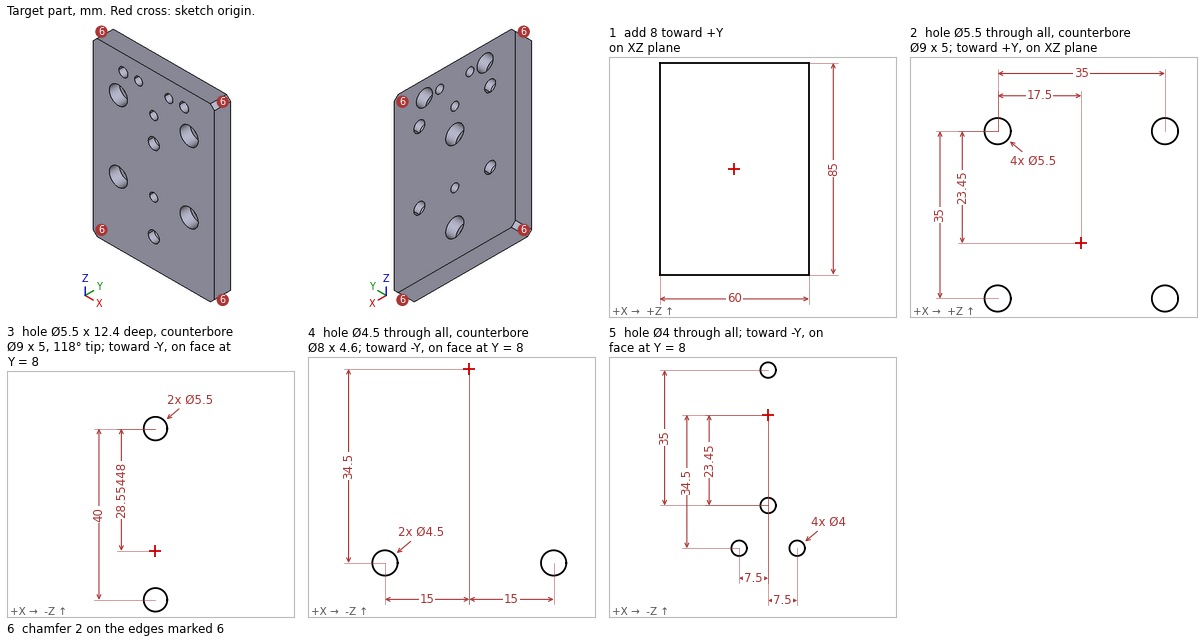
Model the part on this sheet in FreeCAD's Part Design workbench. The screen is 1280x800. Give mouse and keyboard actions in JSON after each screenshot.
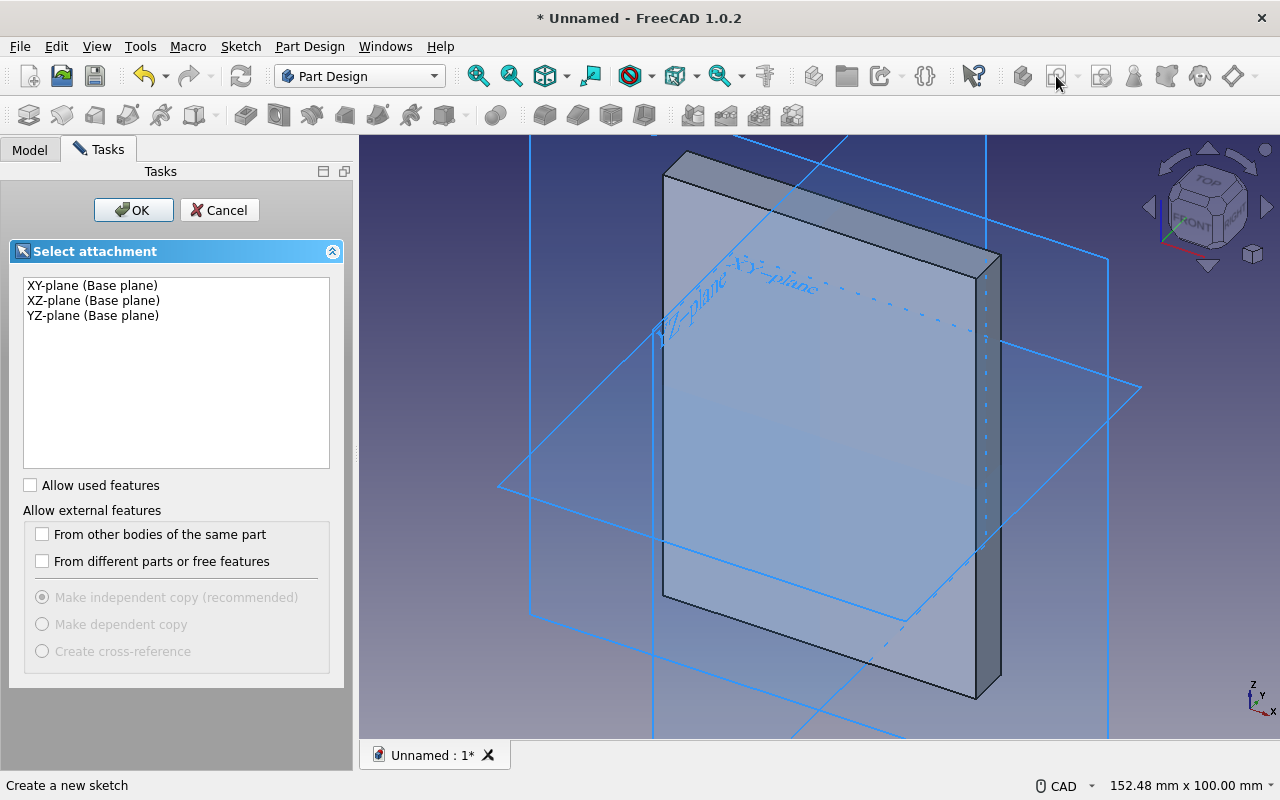
{"action": "left_click", "coordinate": [84, 300]}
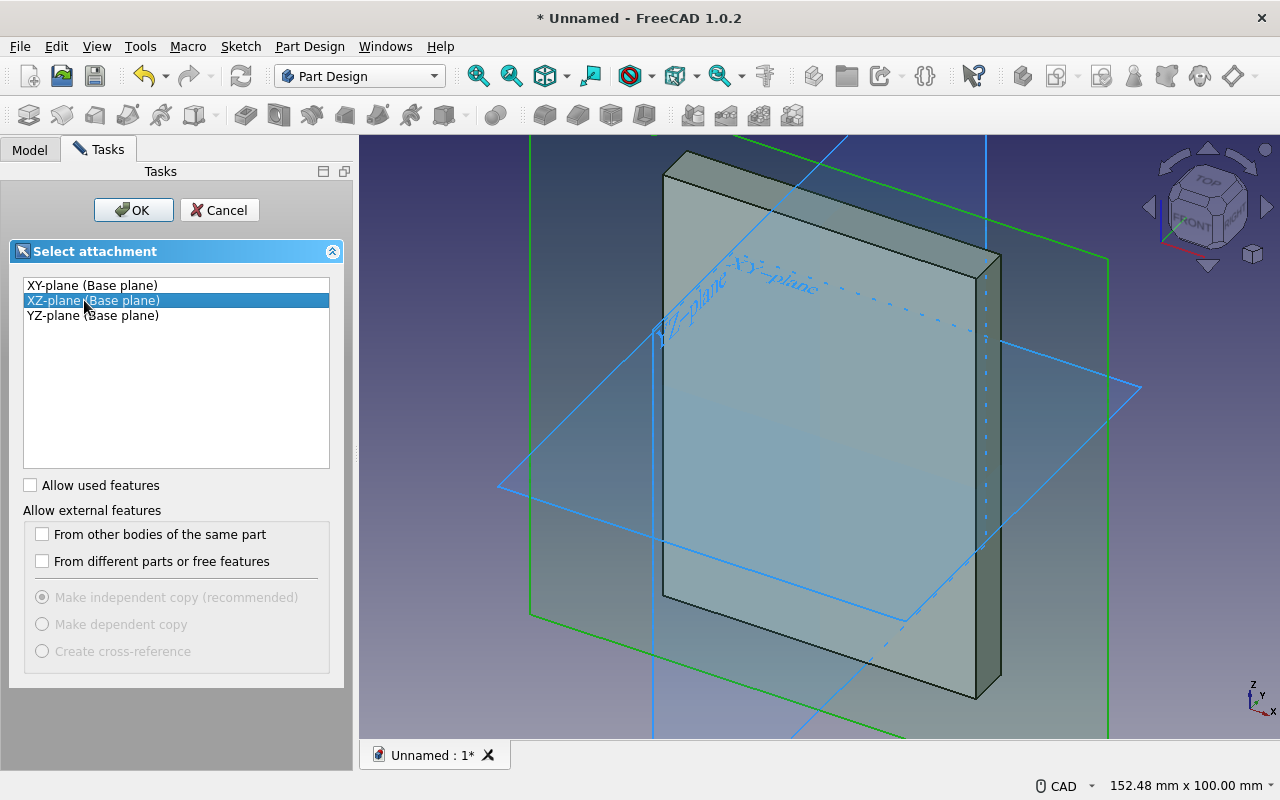
{"action": "left_click", "coordinate": [134, 210]}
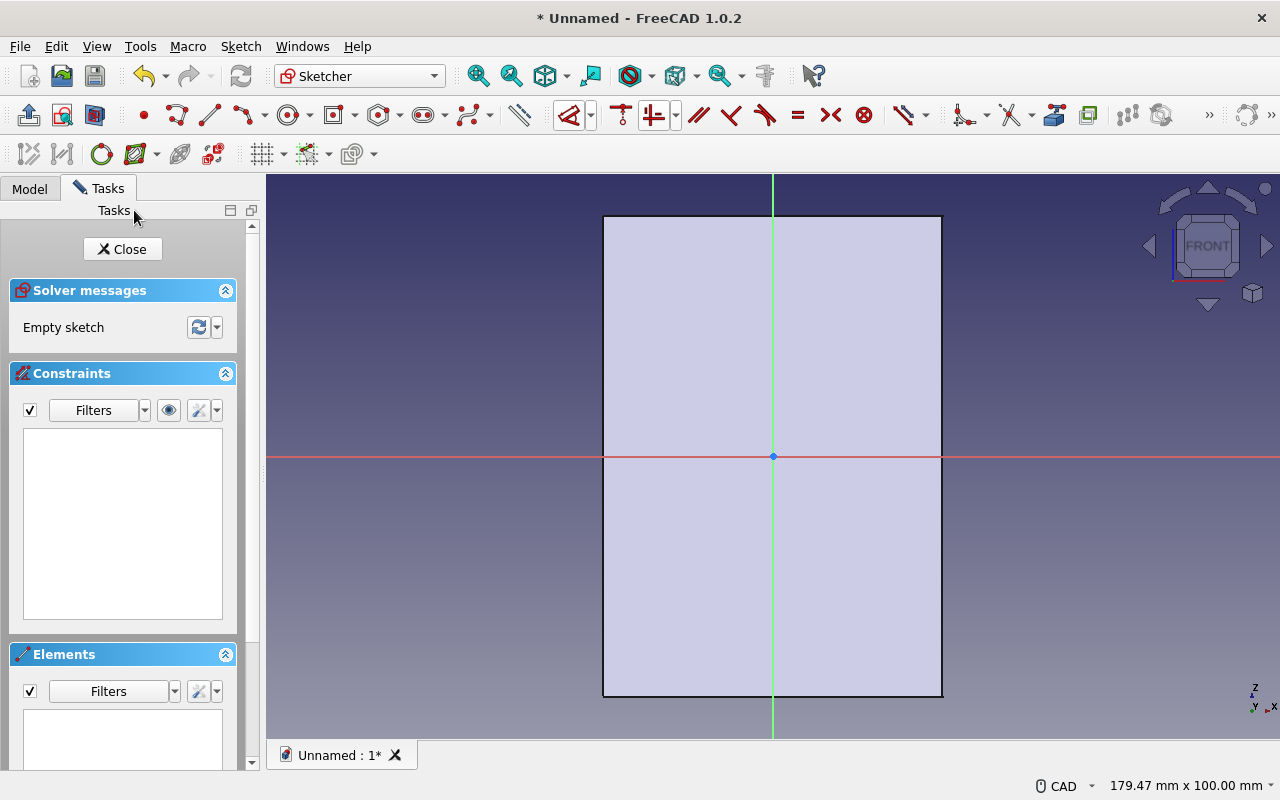
{"action": "scroll", "coordinate": [912, 355], "scroll_direction": "up", "scroll_amount": 2}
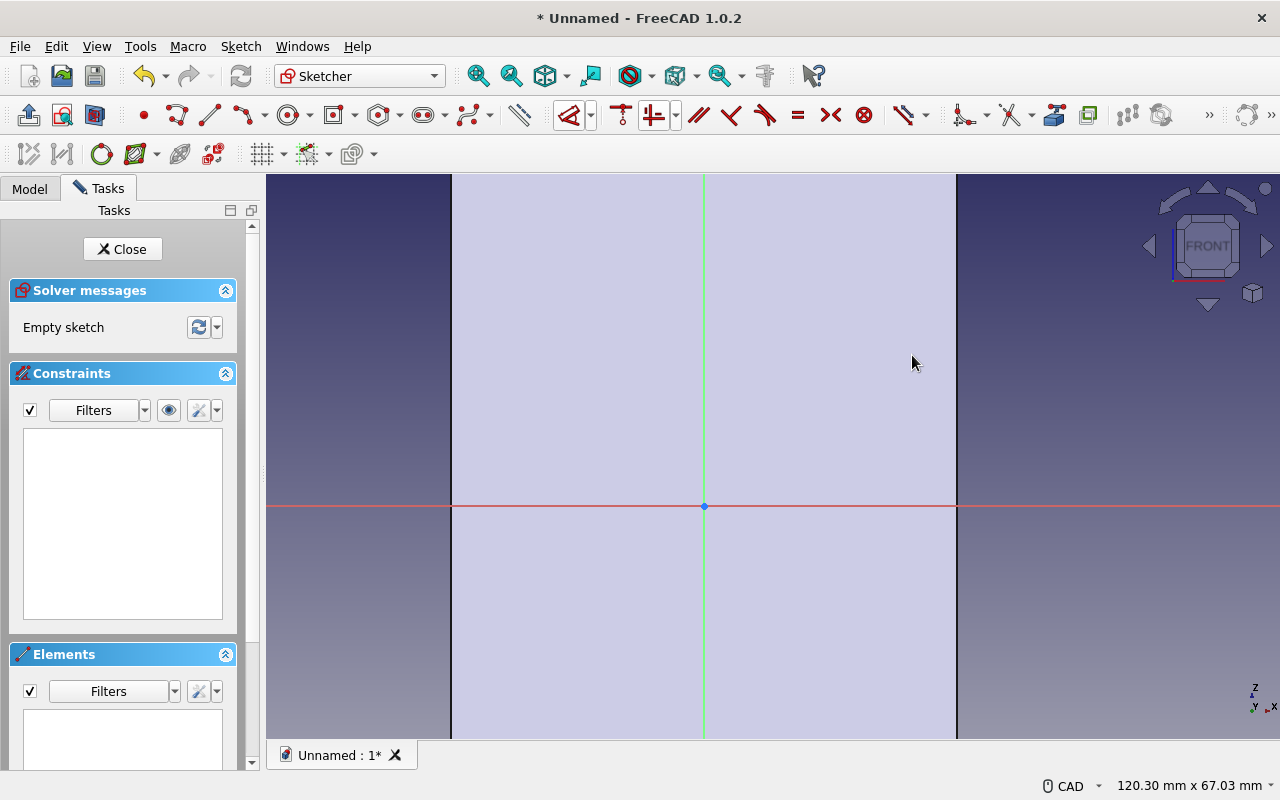
{"action": "key", "text": "g c"}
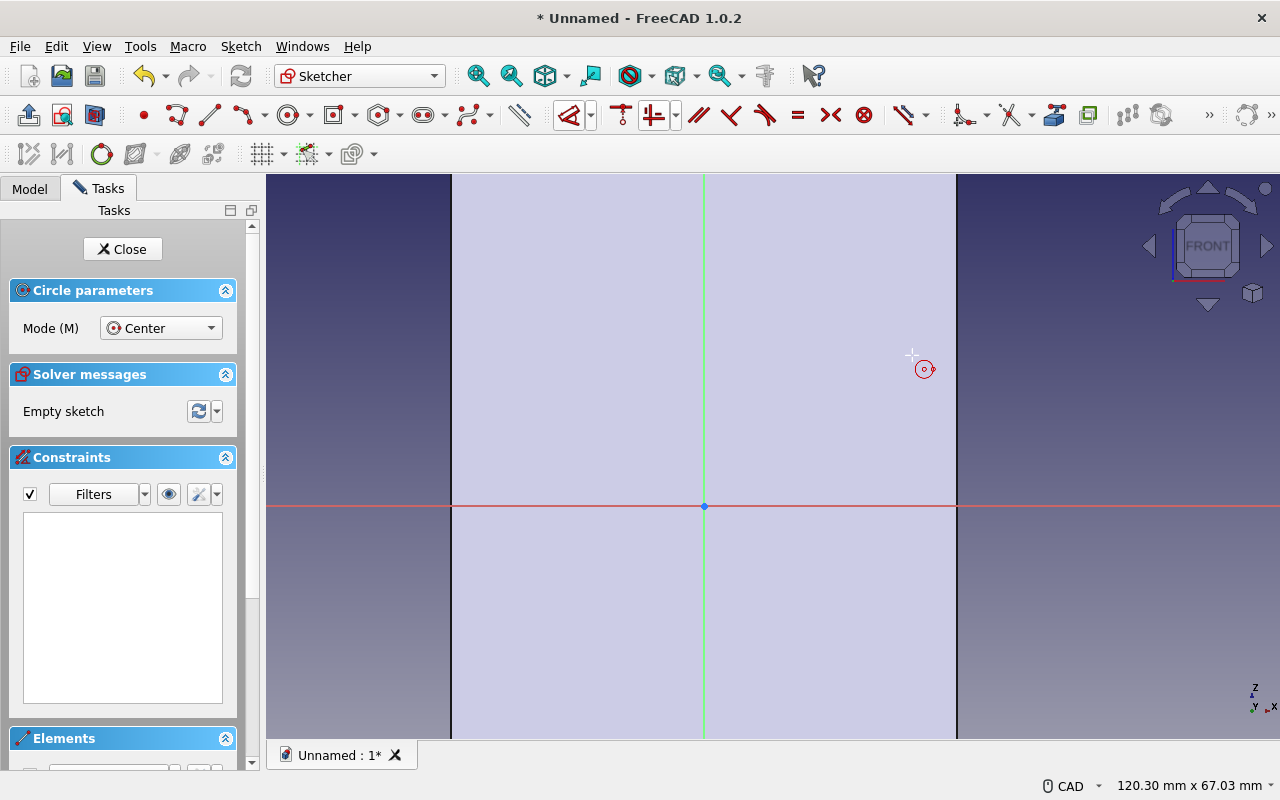
{"action": "left_click", "coordinate": [557, 309]}
{"action": "left_click", "coordinate": [573, 292]}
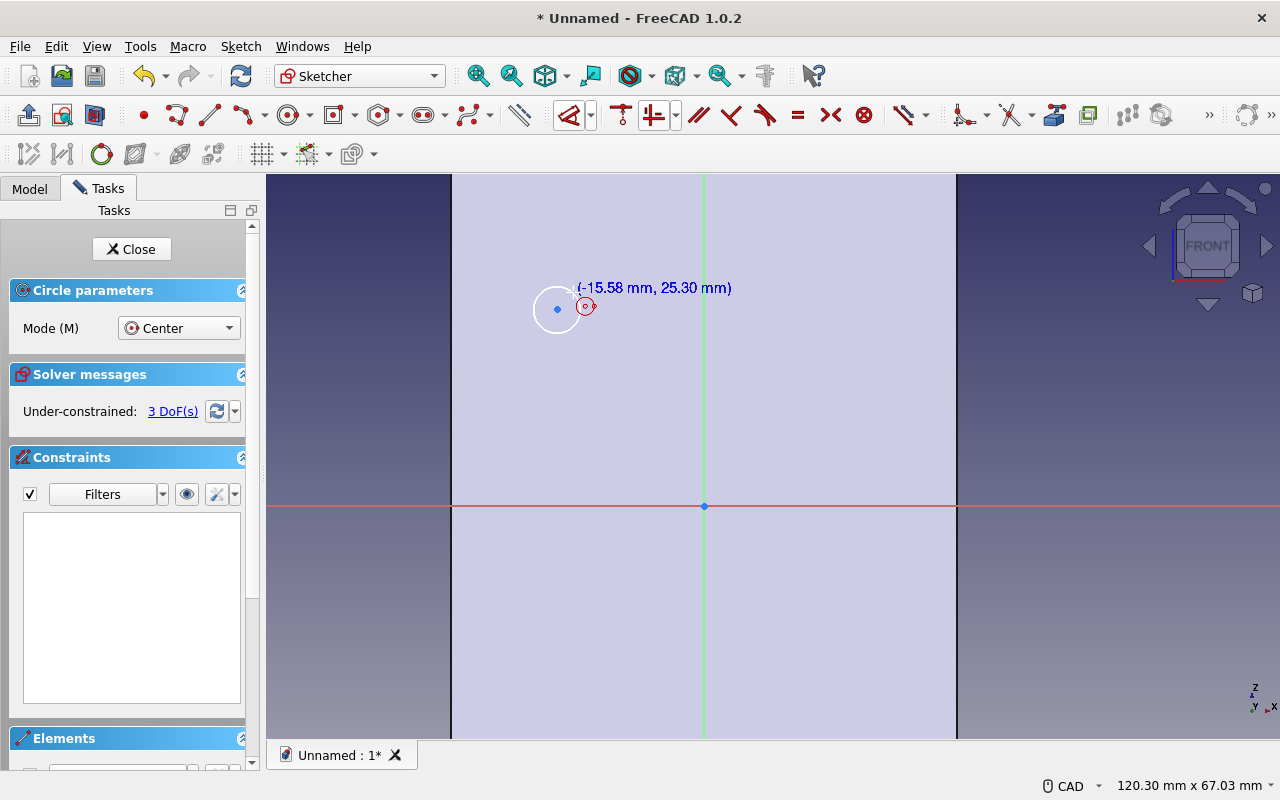
{"action": "left_click", "coordinate": [852, 309]}
{"action": "left_click", "coordinate": [868, 292]}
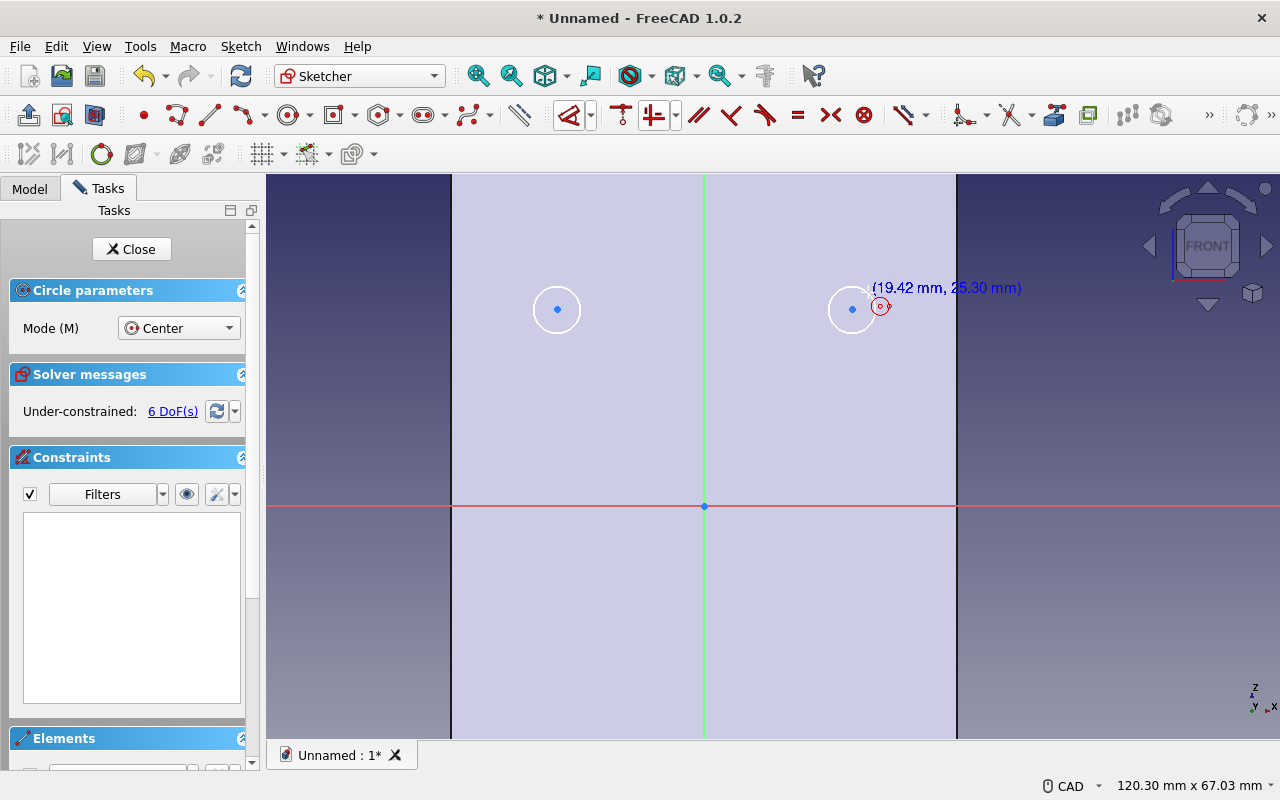
{"action": "left_click", "coordinate": [557, 604]}
{"action": "left_click", "coordinate": [573, 587]}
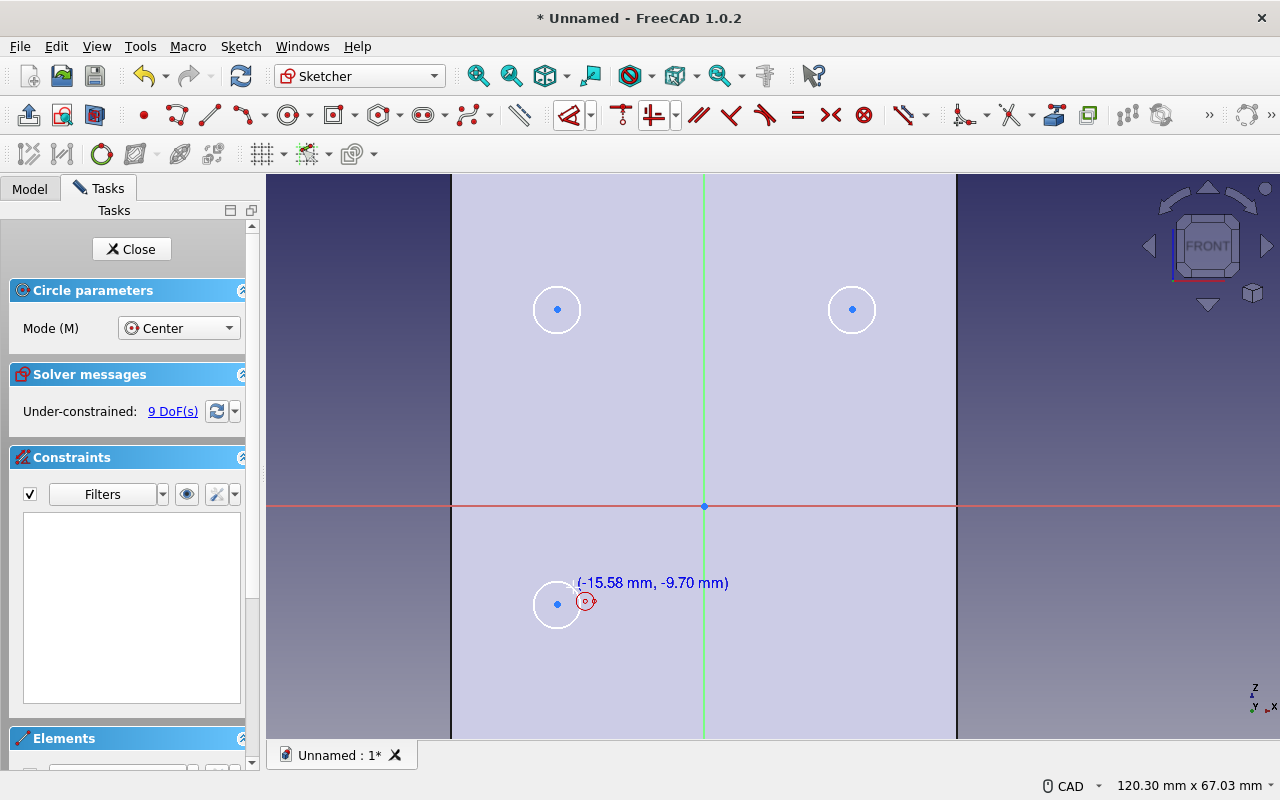
{"action": "left_click", "coordinate": [852, 604]}
{"action": "left_click", "coordinate": [868, 587]}
{"action": "key", "text": "Escape"}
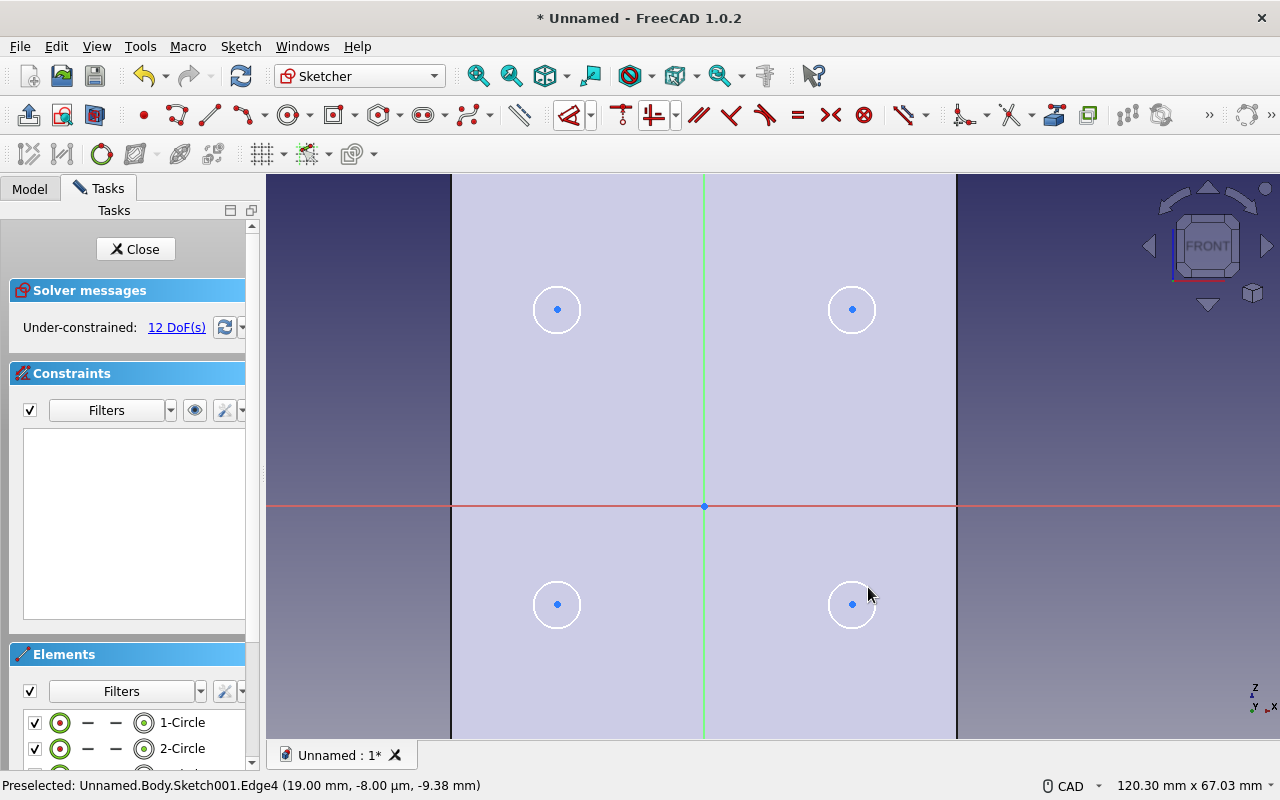
{"action": "left_click", "coordinate": [573, 293]}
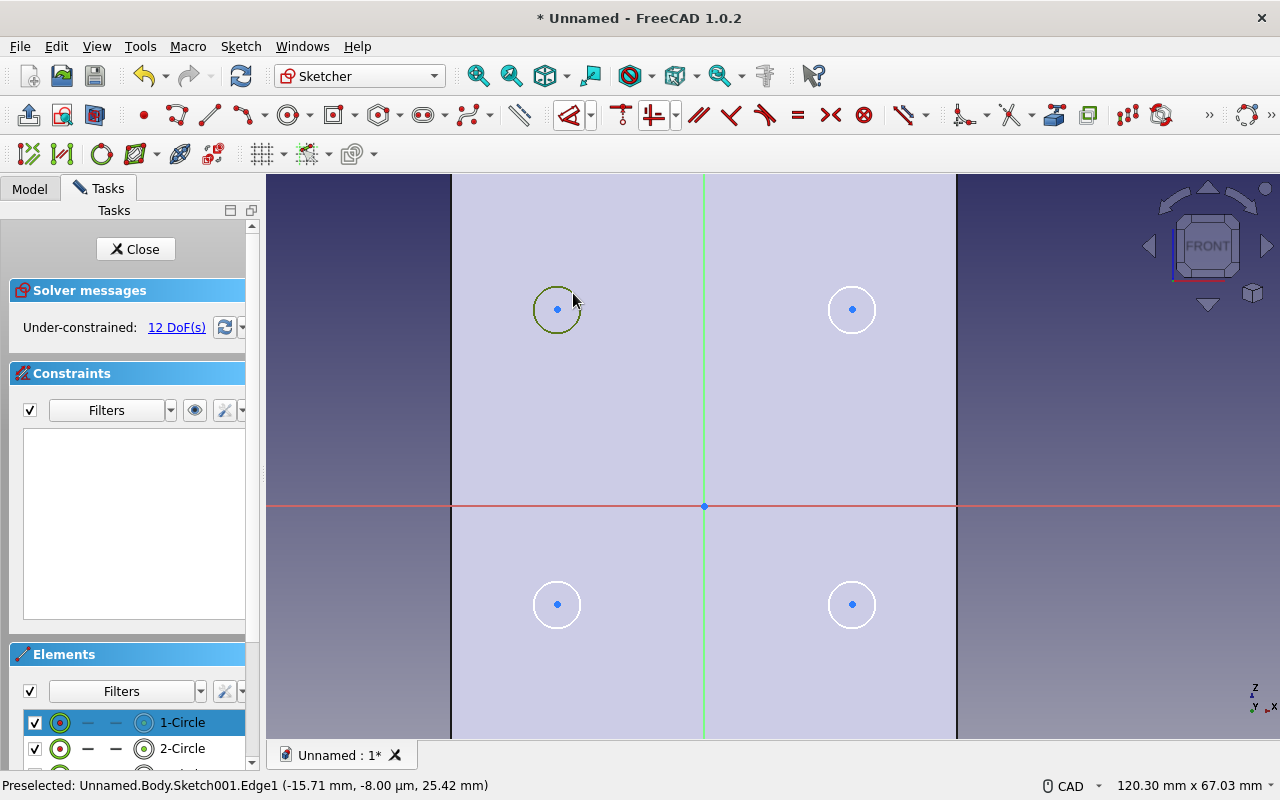
{"action": "left_click", "coordinate": [868, 293]}